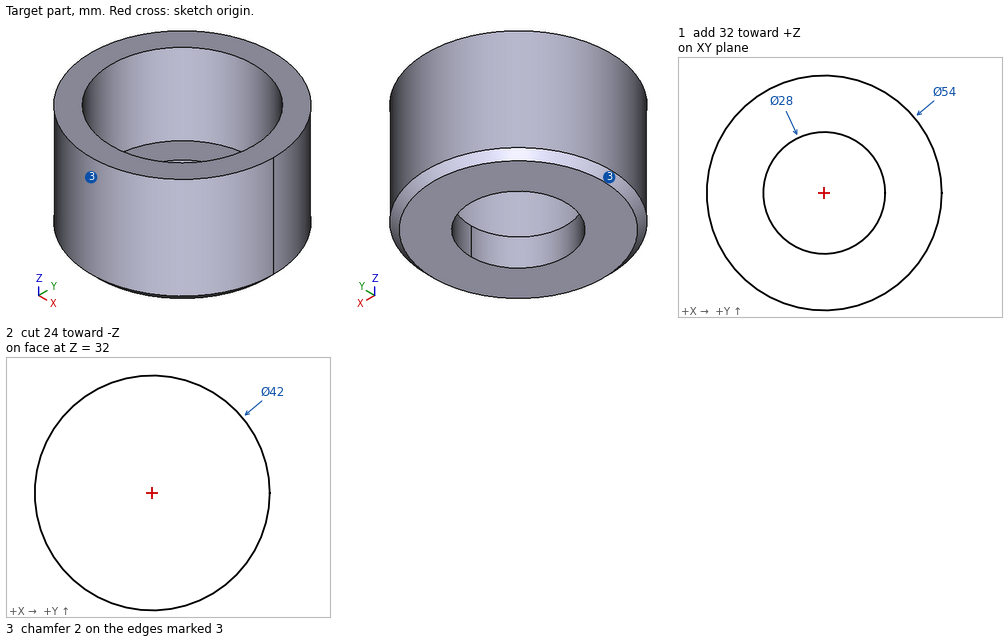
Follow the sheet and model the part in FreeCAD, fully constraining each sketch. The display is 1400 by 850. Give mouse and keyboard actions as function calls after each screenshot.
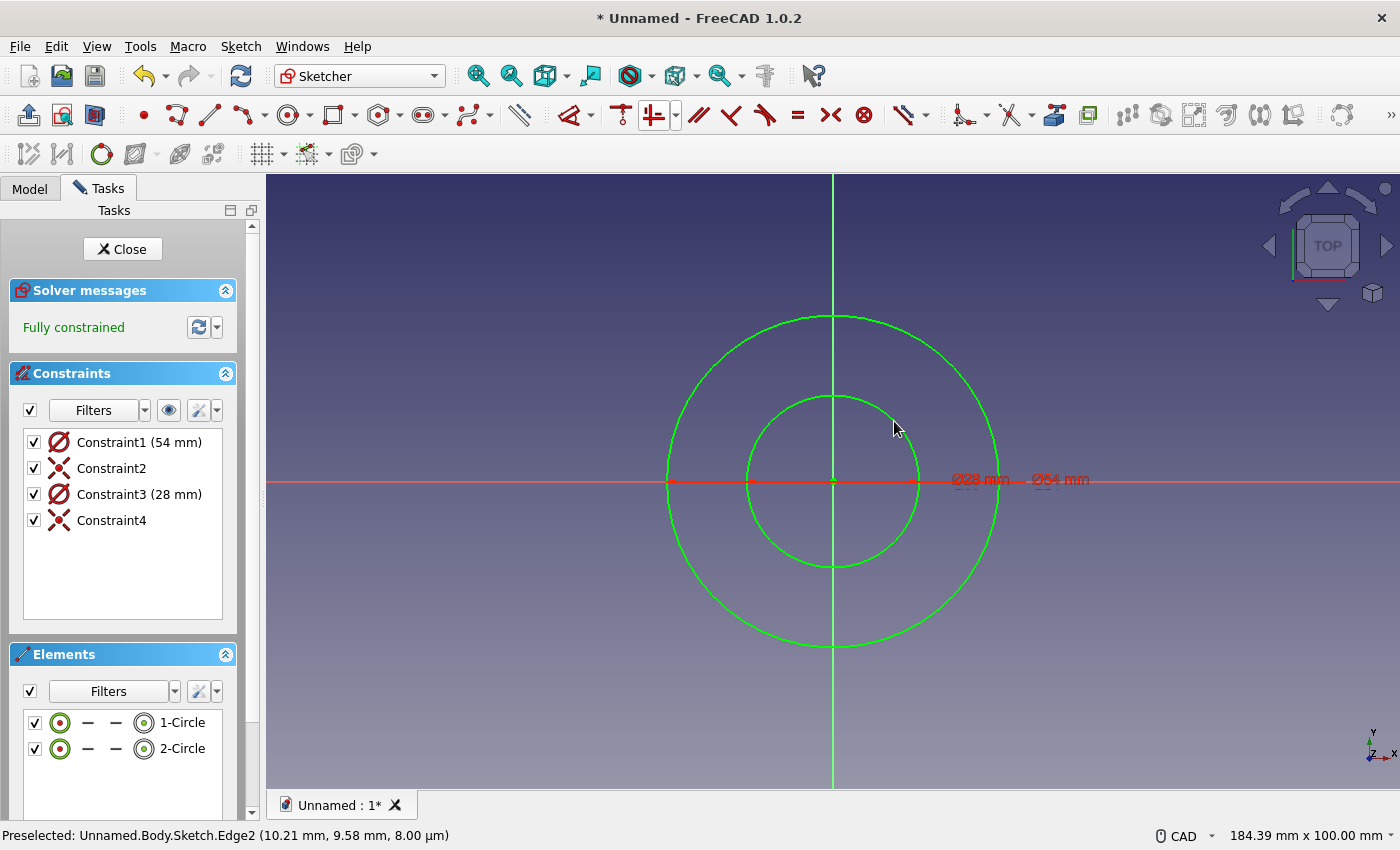
click(123, 249)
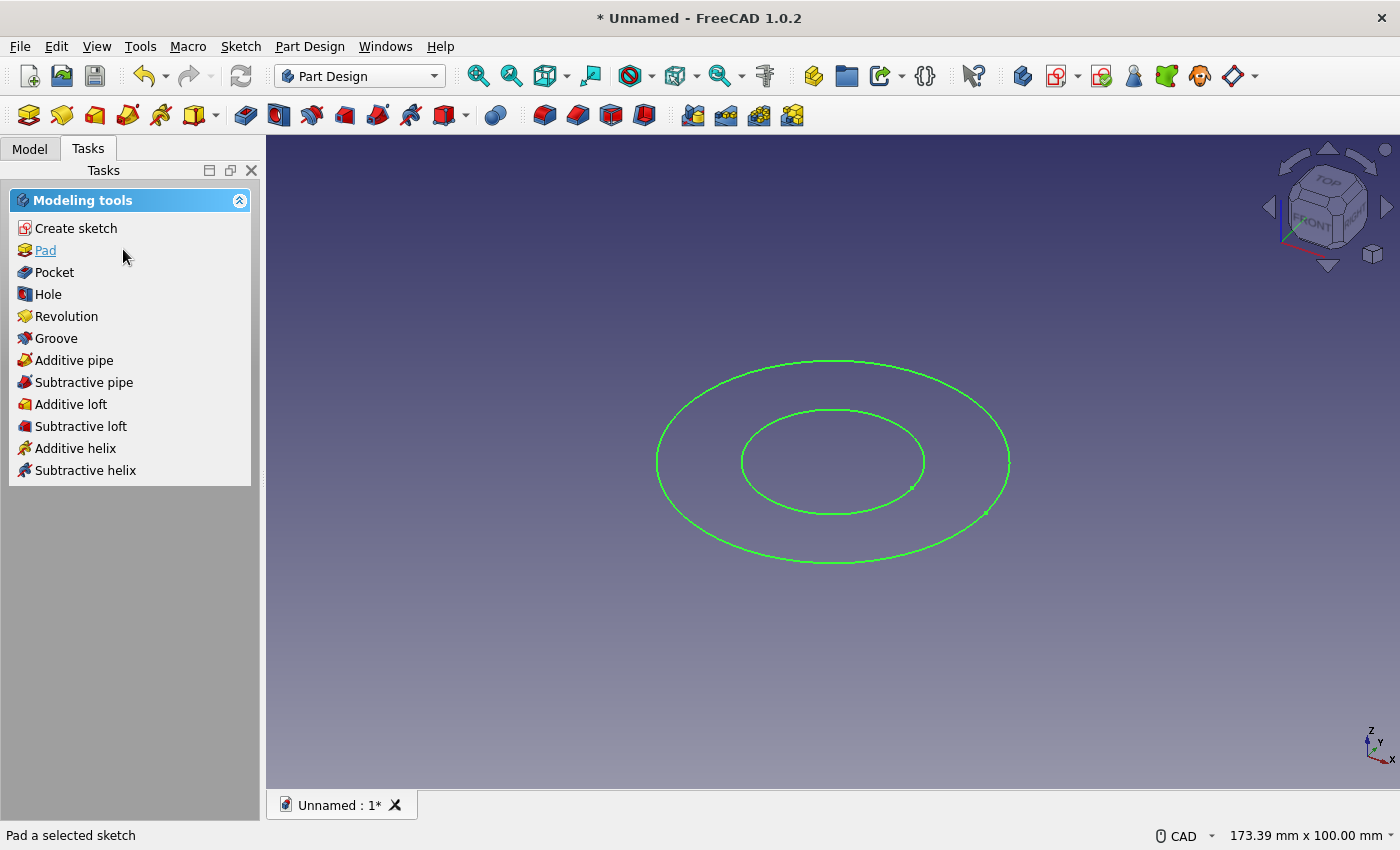
click(29, 116)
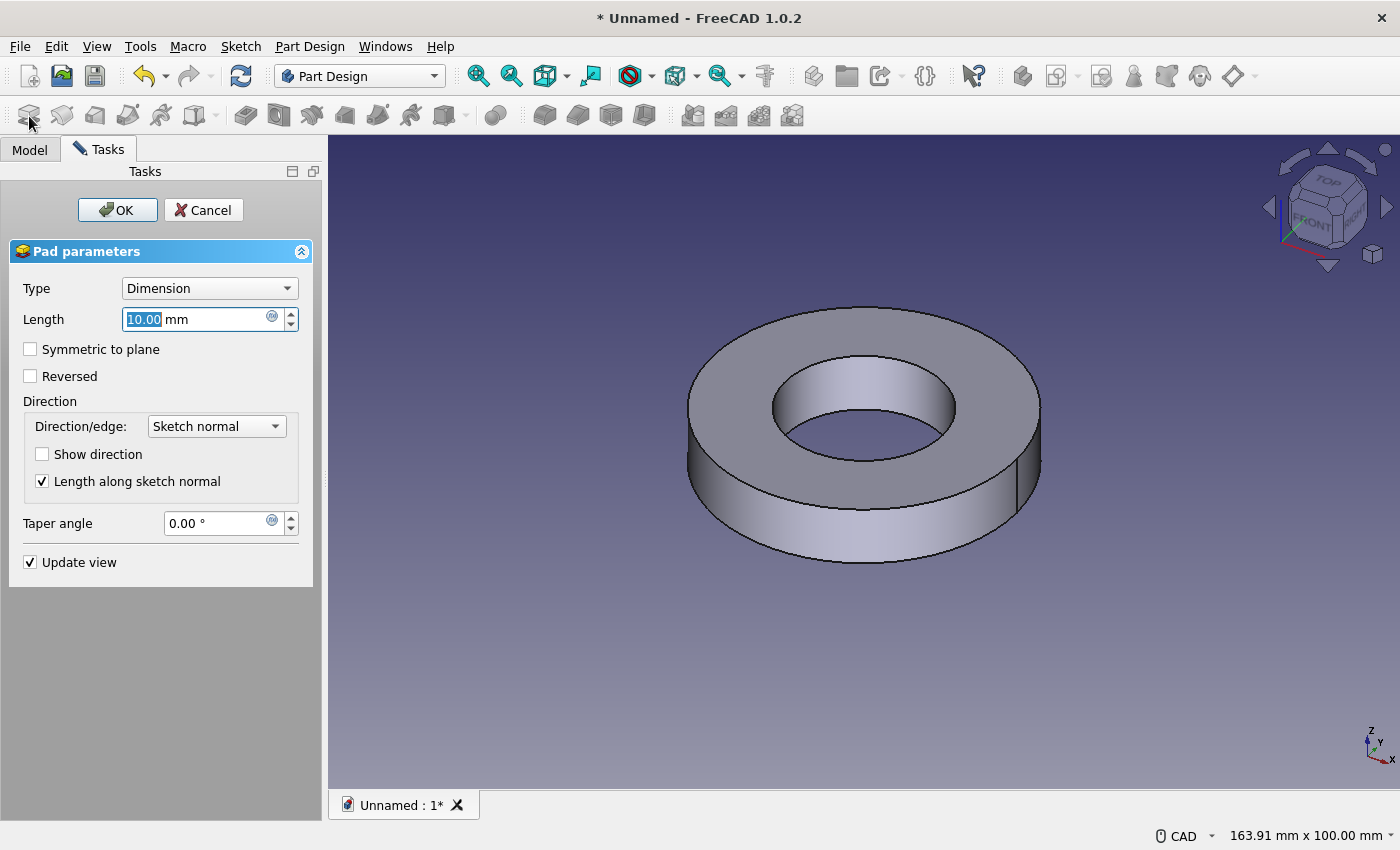
text(32)
key(Tab)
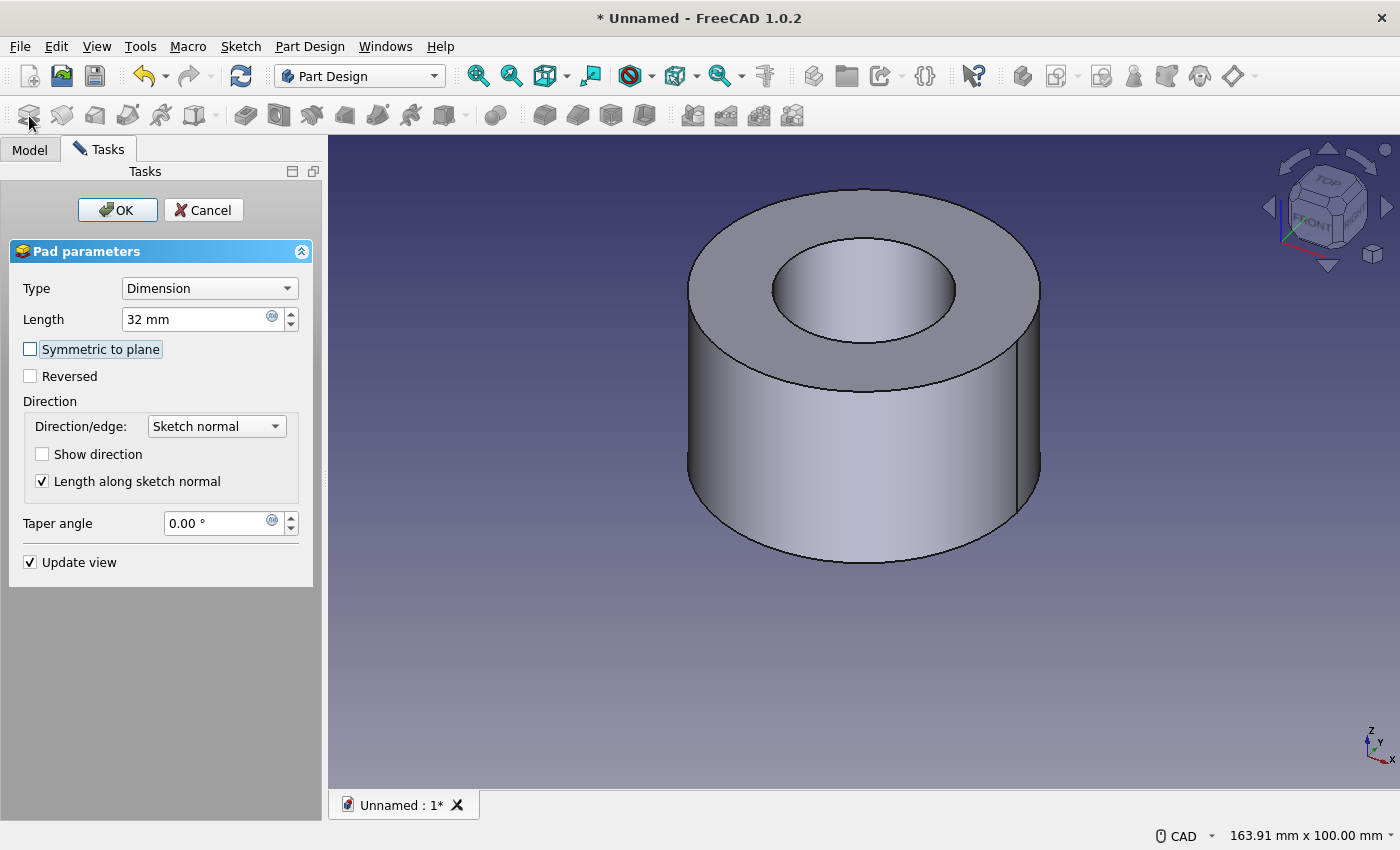
click(118, 210)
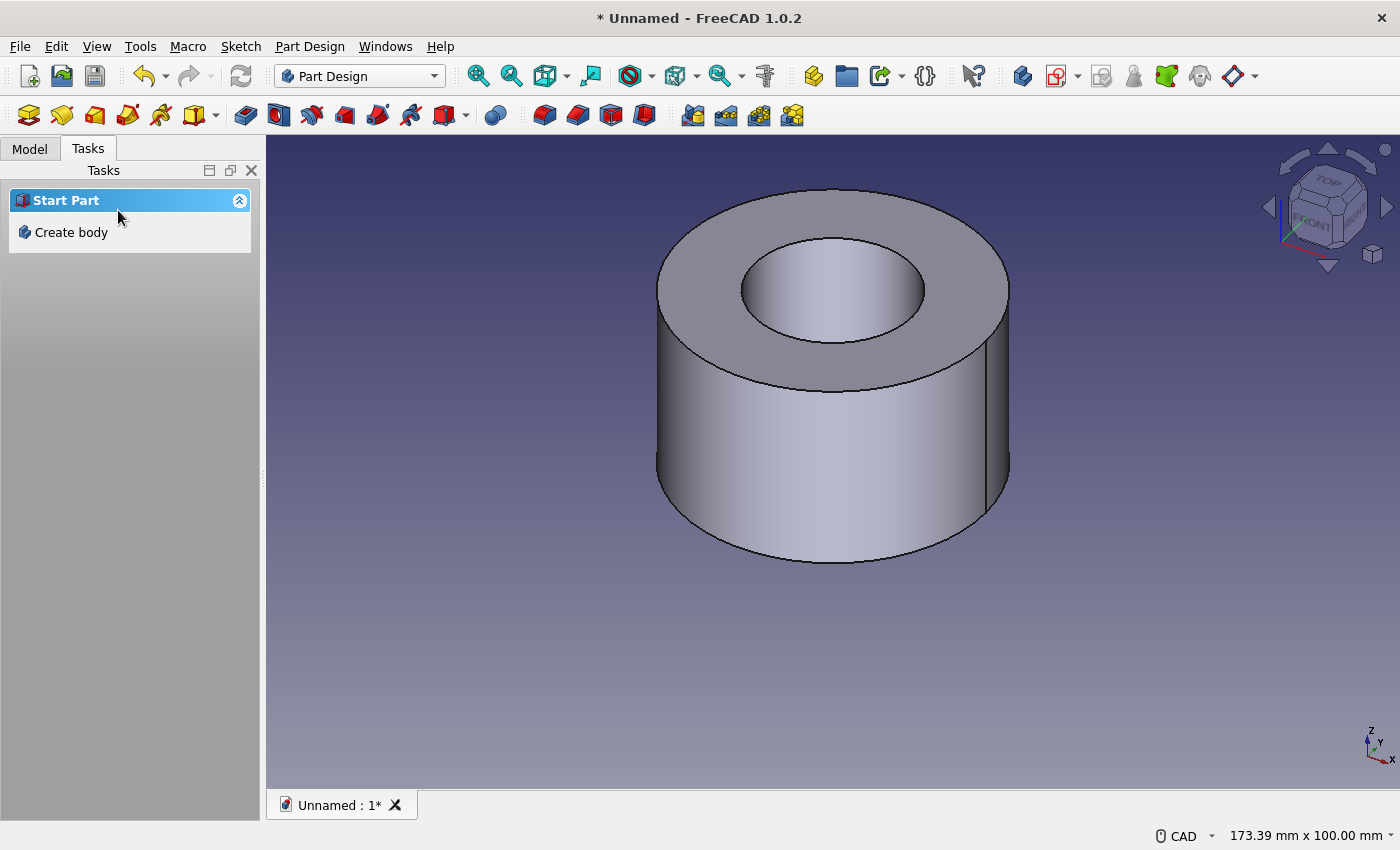
click(695, 311)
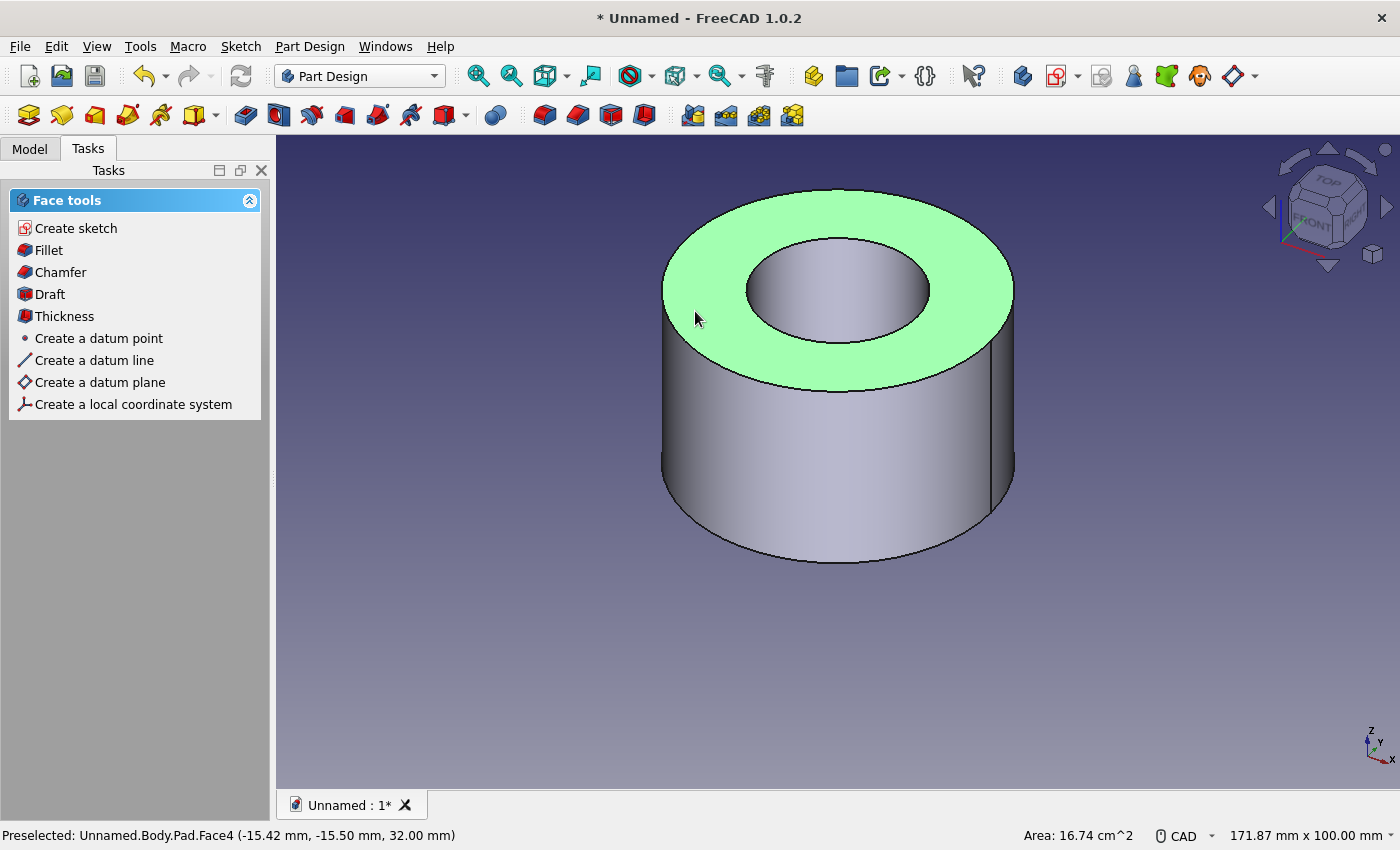
click(1056, 76)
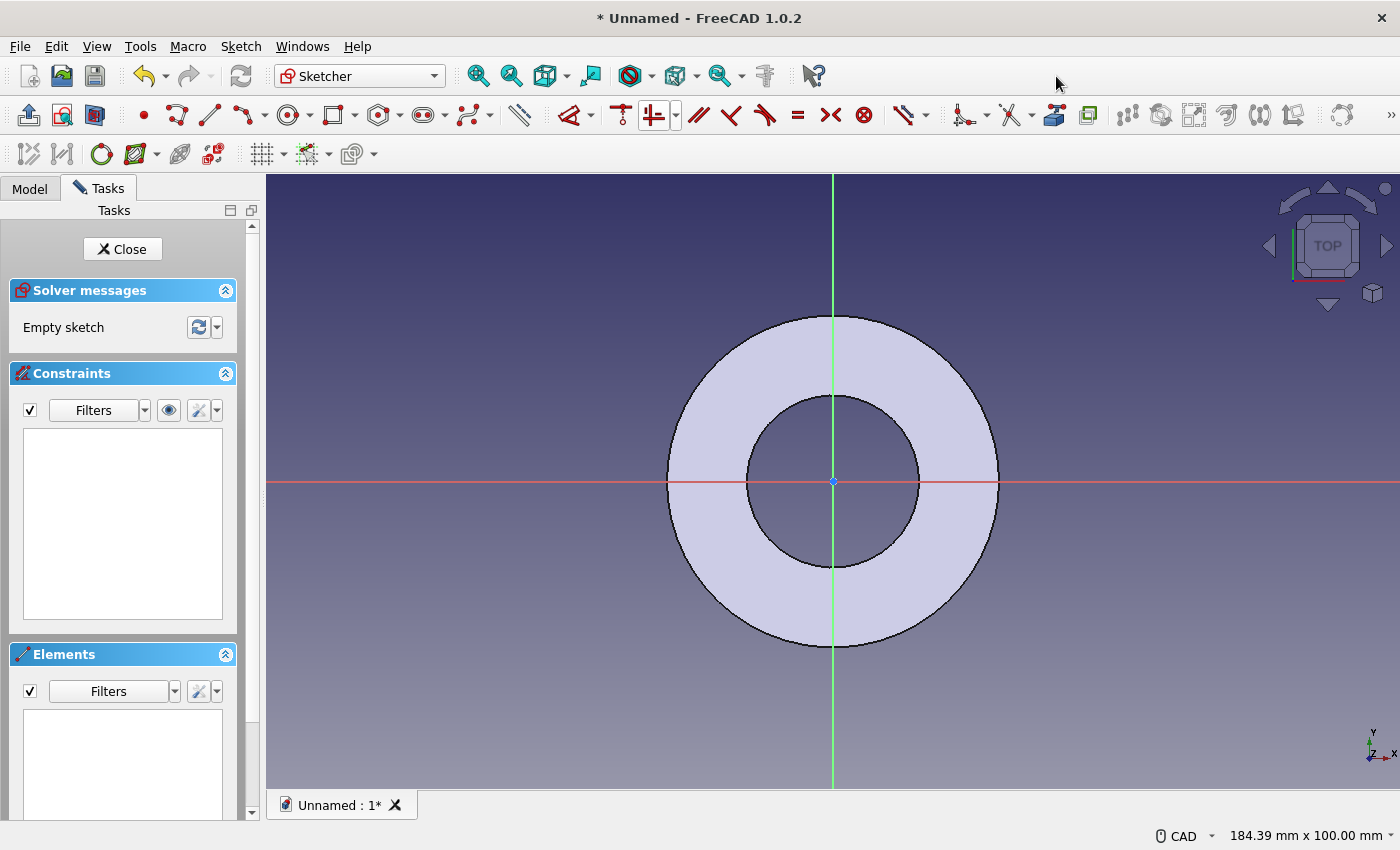
scroll(972, 482, up, 2)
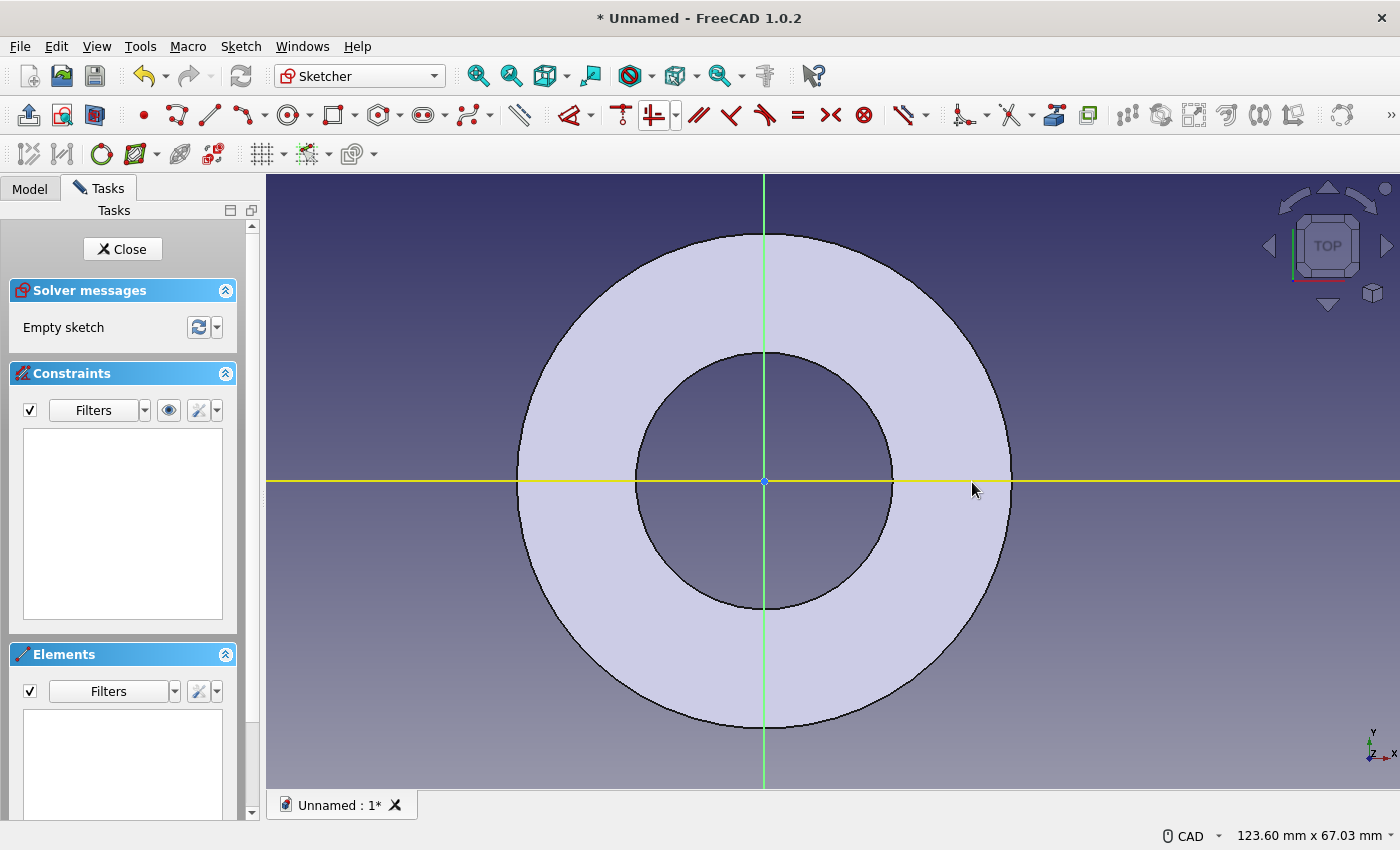
key(g)
key(c)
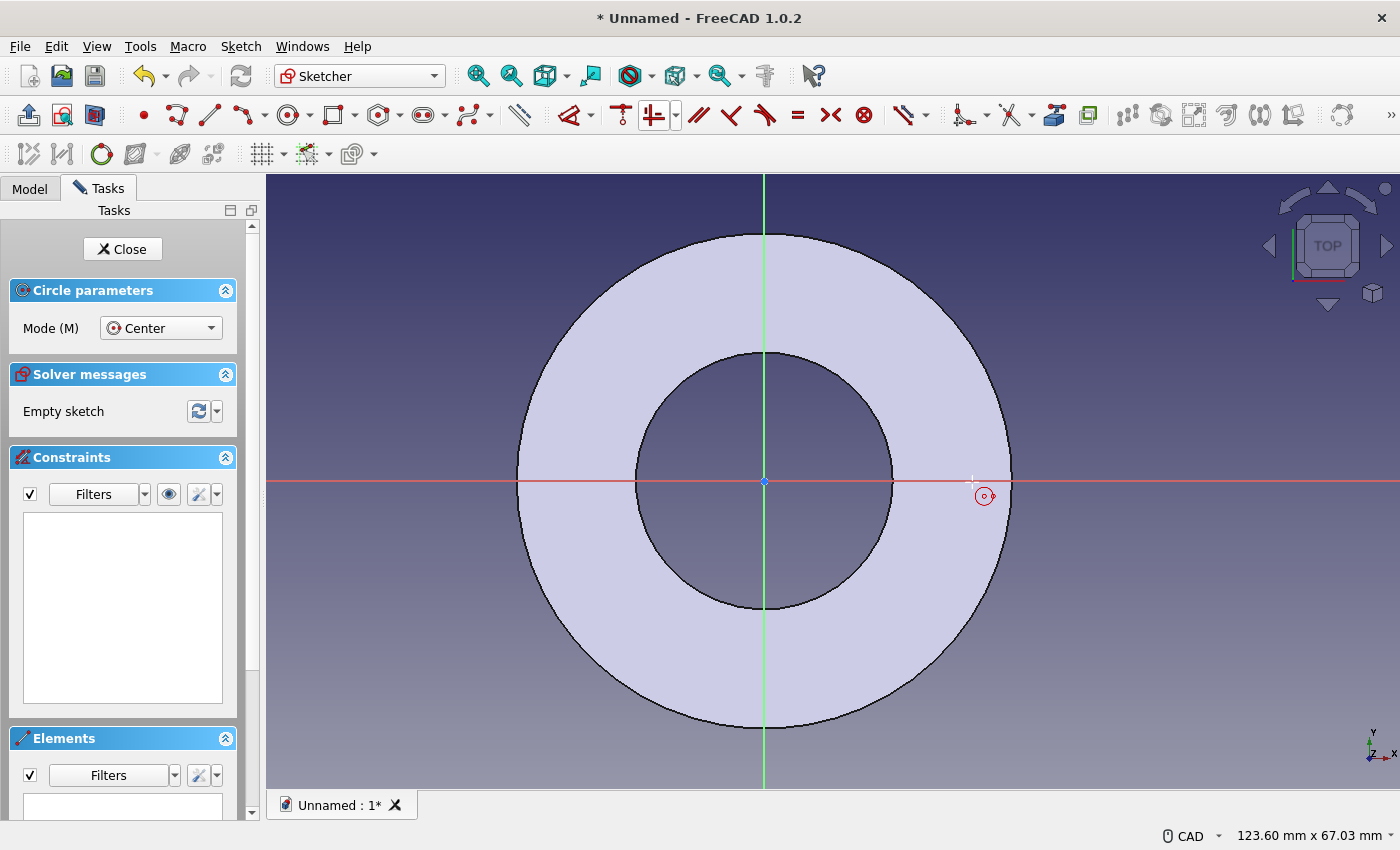
click(764, 481)
move(901, 345)